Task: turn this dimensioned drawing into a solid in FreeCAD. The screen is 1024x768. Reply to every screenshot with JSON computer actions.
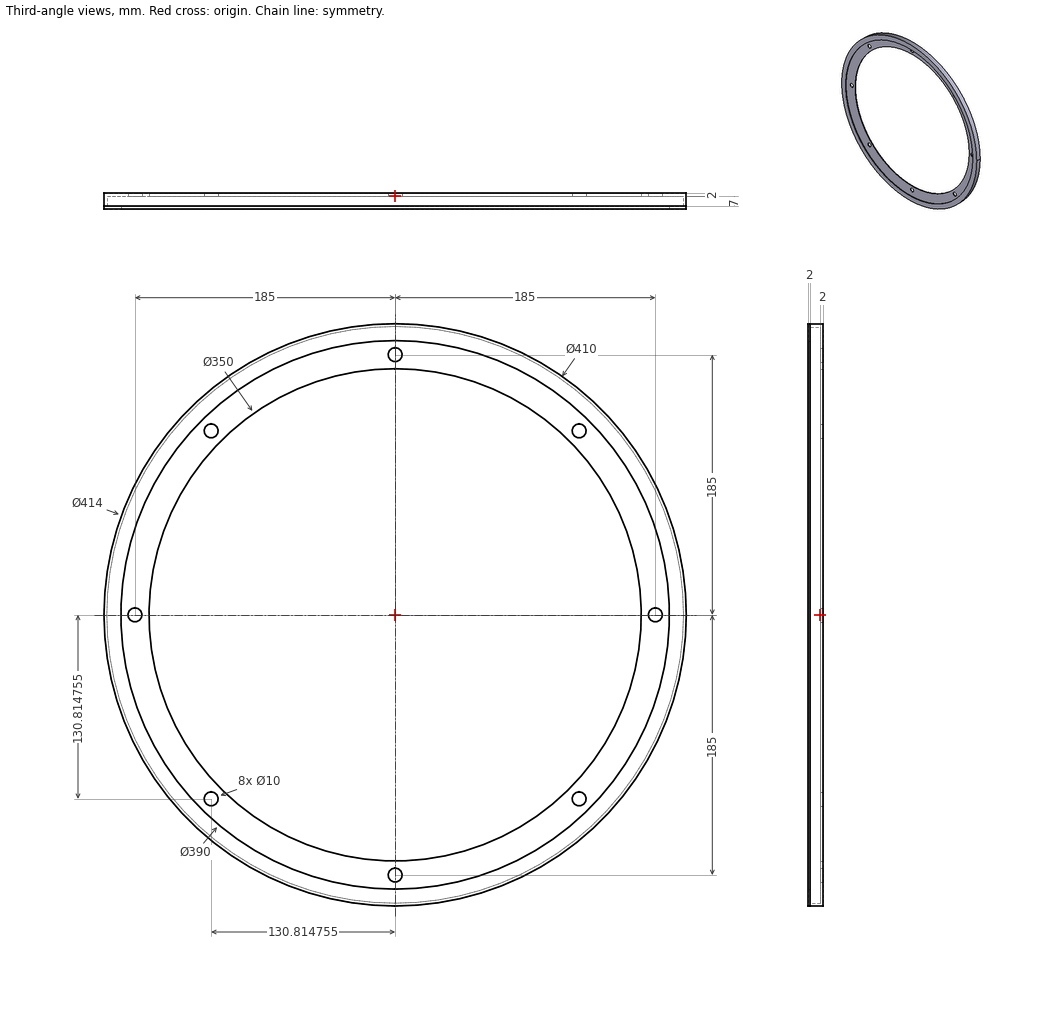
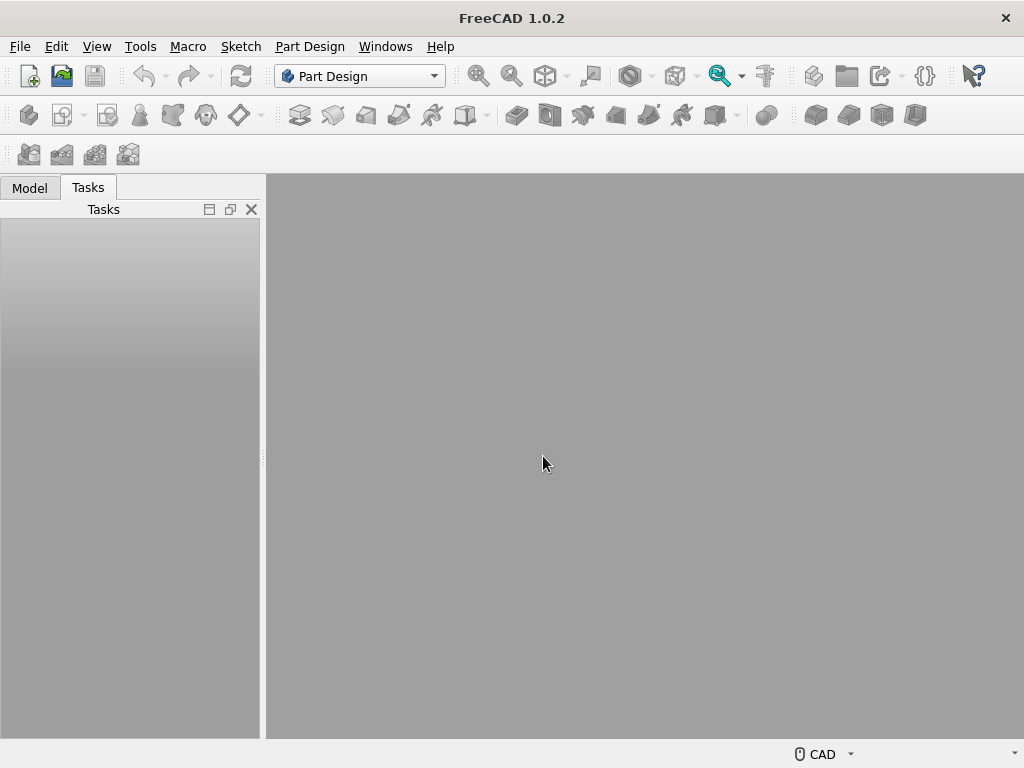
{"action": "left_click", "coordinate": [29, 76]}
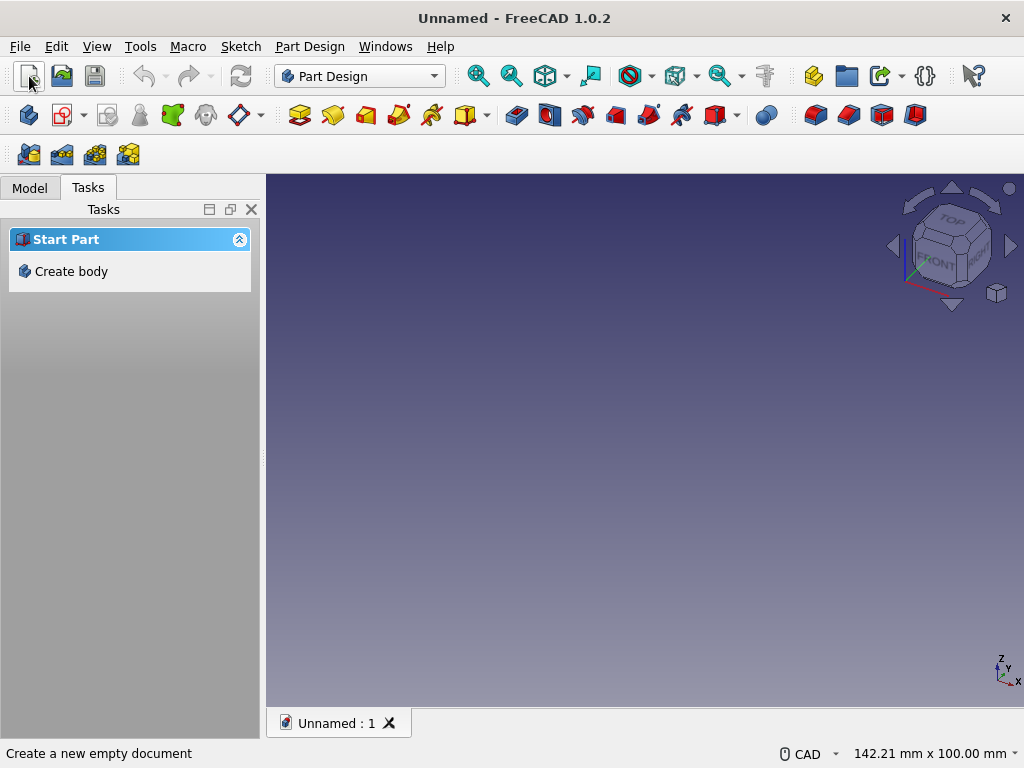
{"action": "left_click", "coordinate": [62, 116]}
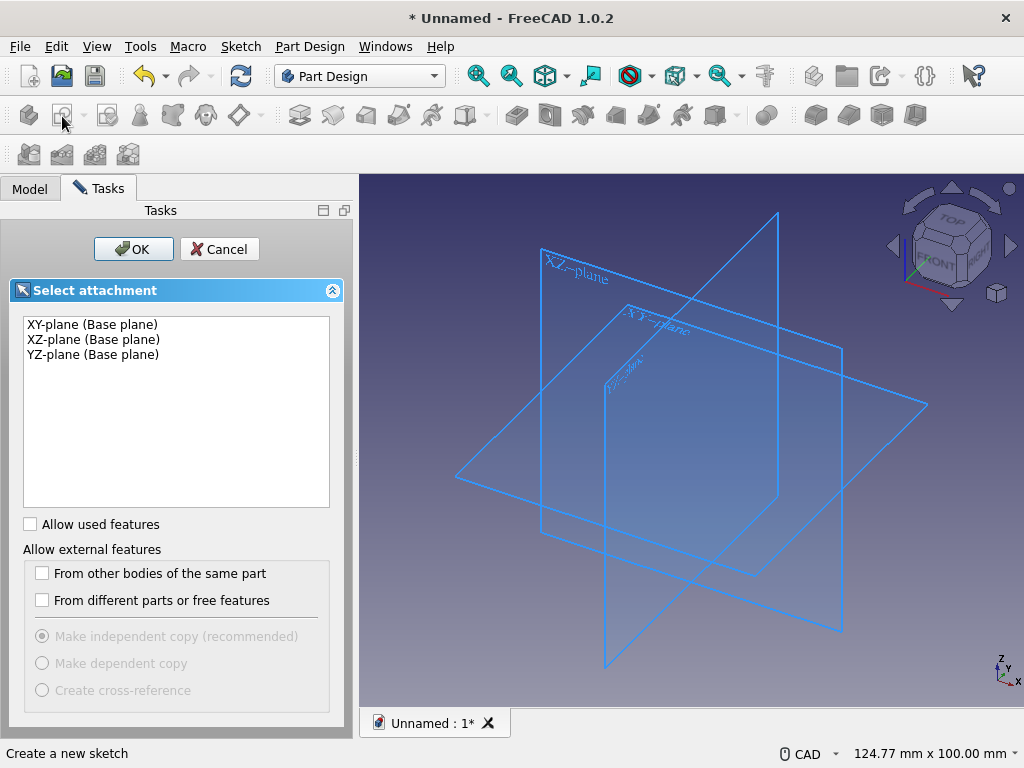
{"action": "left_click", "coordinate": [84, 340]}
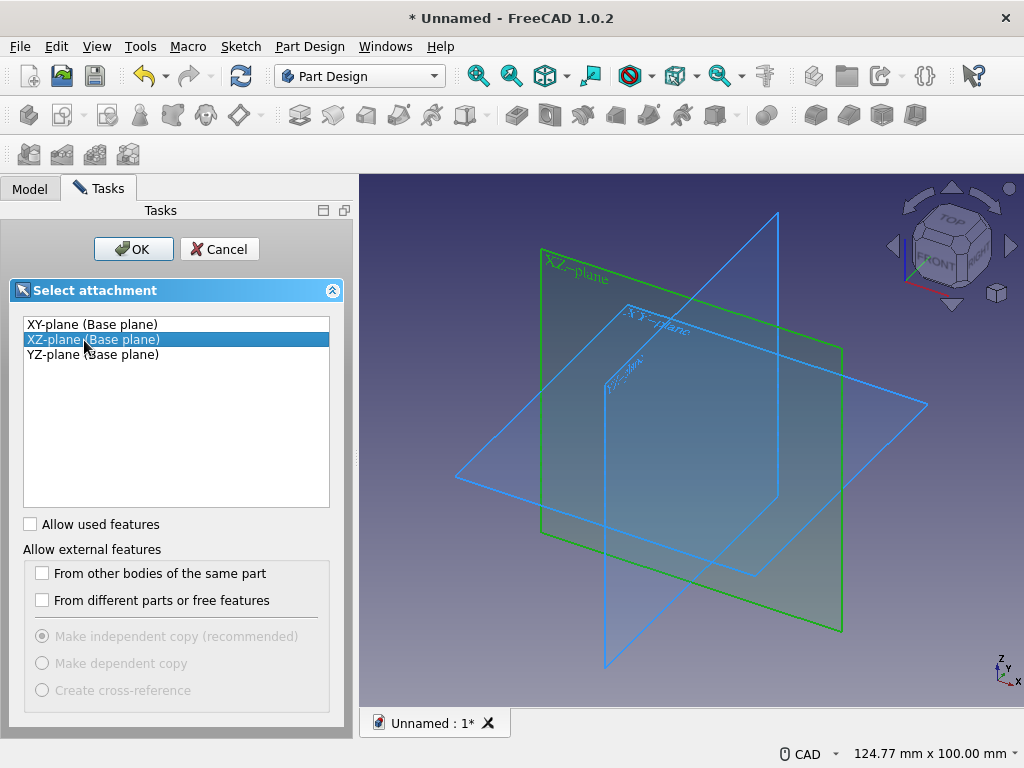
{"action": "left_click", "coordinate": [134, 249]}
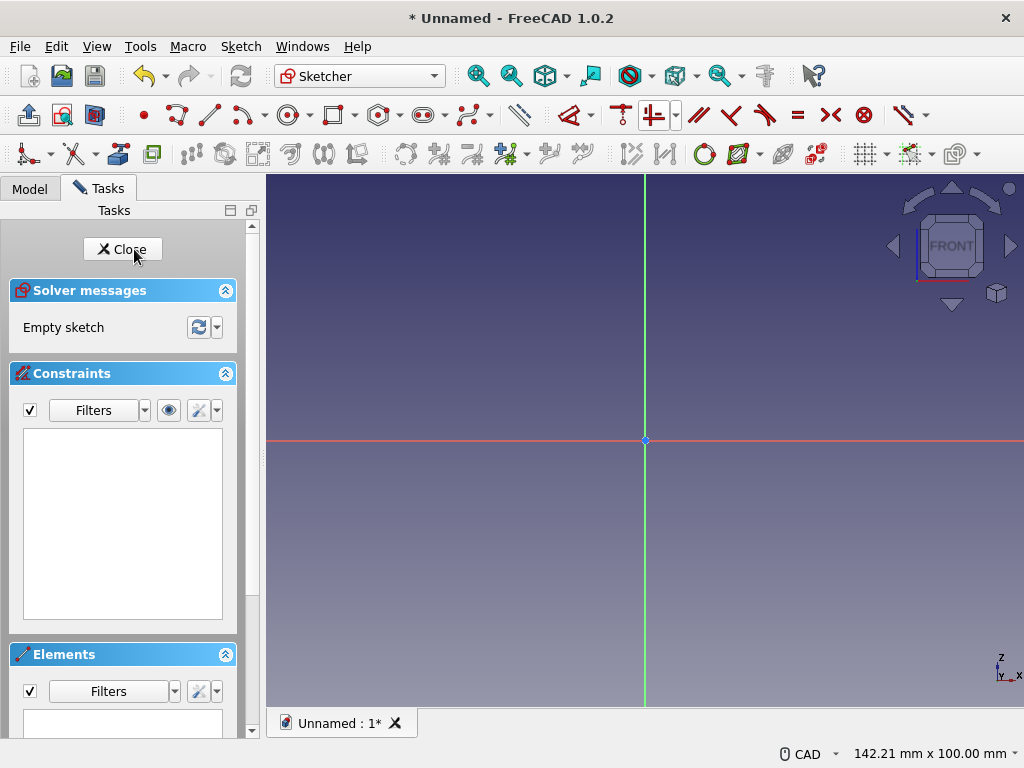
{"action": "scroll", "coordinate": [563, 440], "scroll_direction": "down", "scroll_amount": 9}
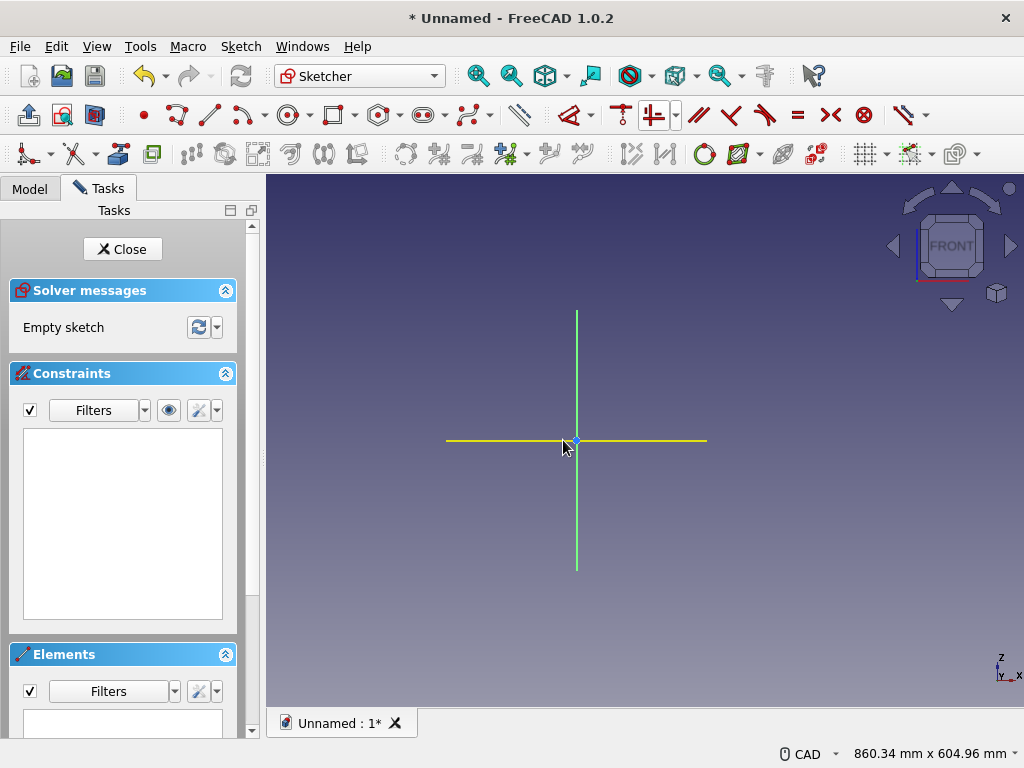
{"action": "left_click", "coordinate": [288, 116]}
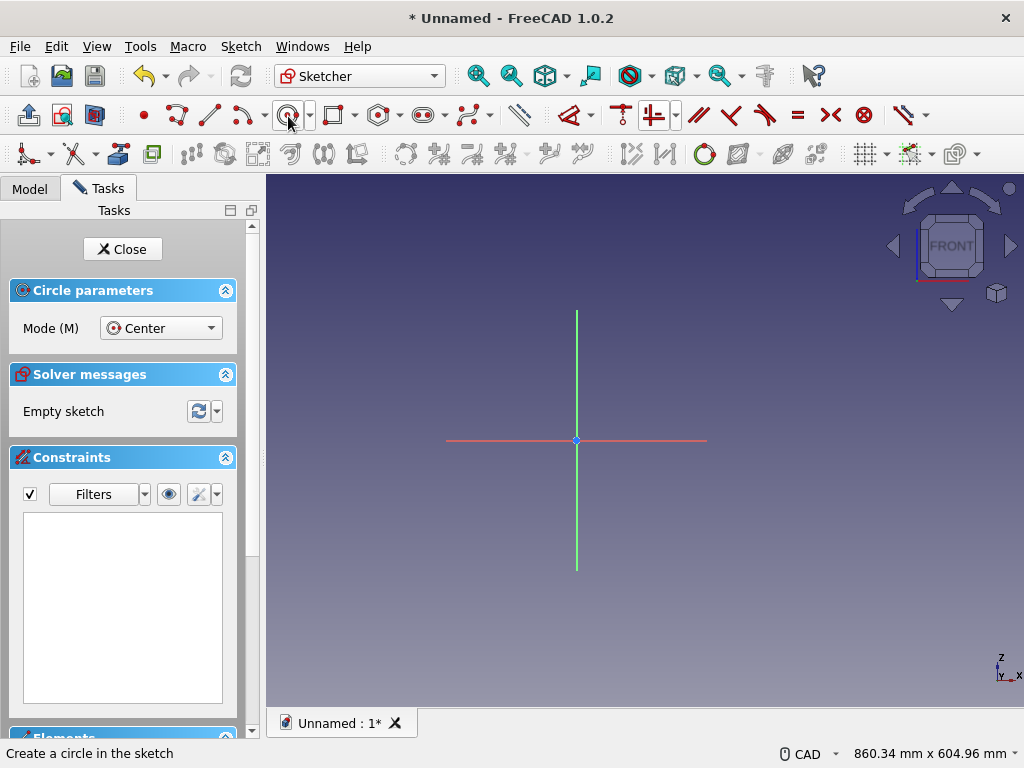
{"action": "left_click", "coordinate": [577, 440]}
{"action": "mouse_move", "coordinate": [705, 313]}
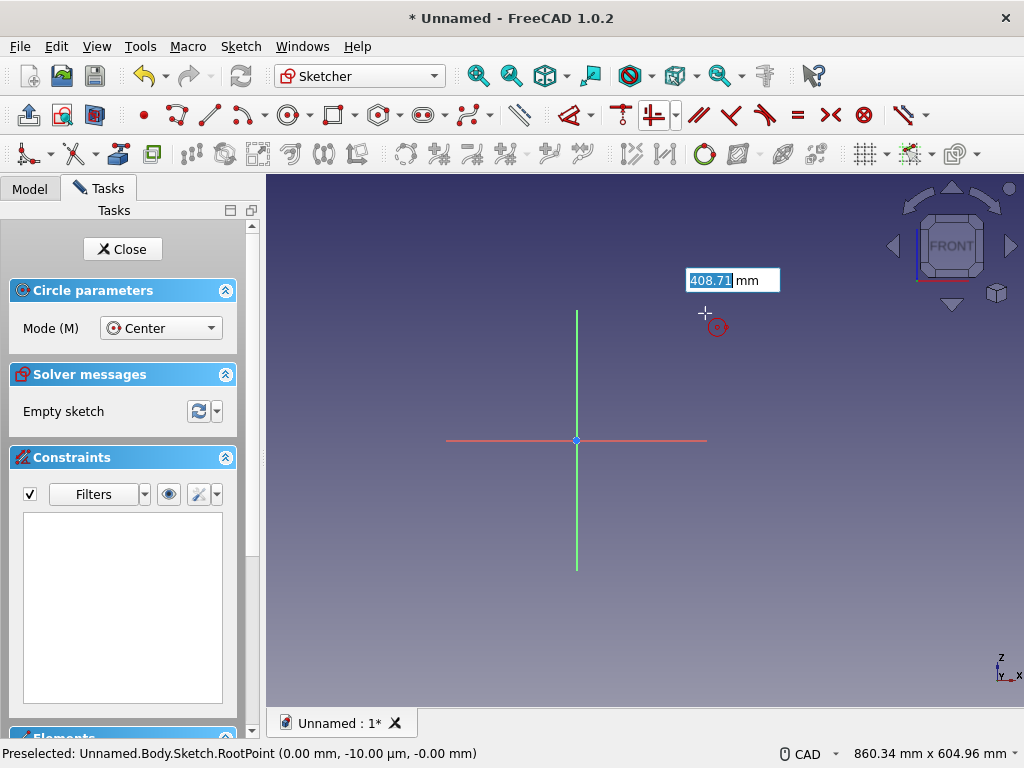
{"action": "type", "text": "410"}
{"action": "key", "text": "Return"}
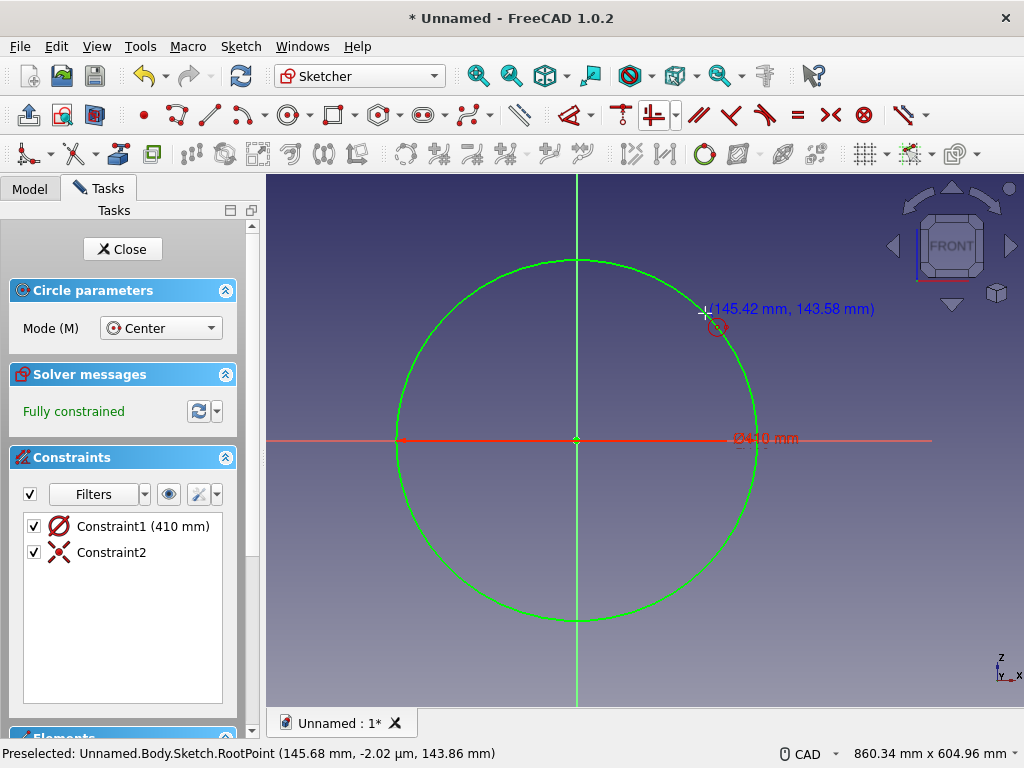
{"action": "scroll", "coordinate": [462, 556], "scroll_direction": "up", "scroll_amount": 9}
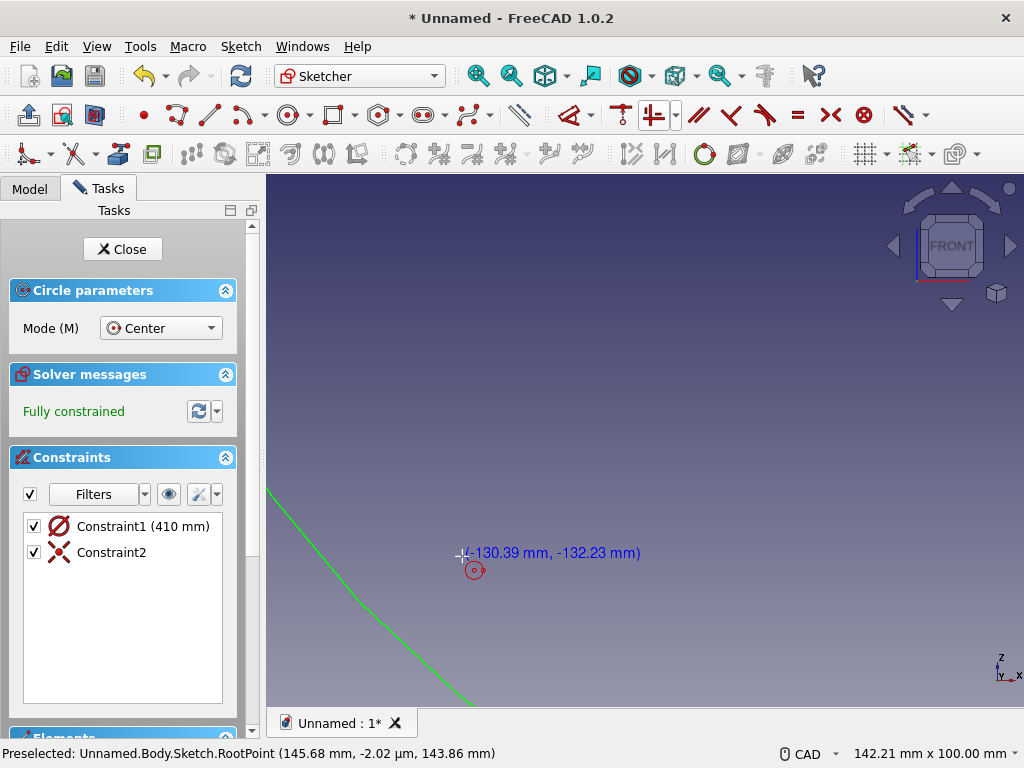
{"action": "scroll", "coordinate": [462, 557], "scroll_direction": "down", "scroll_amount": 9}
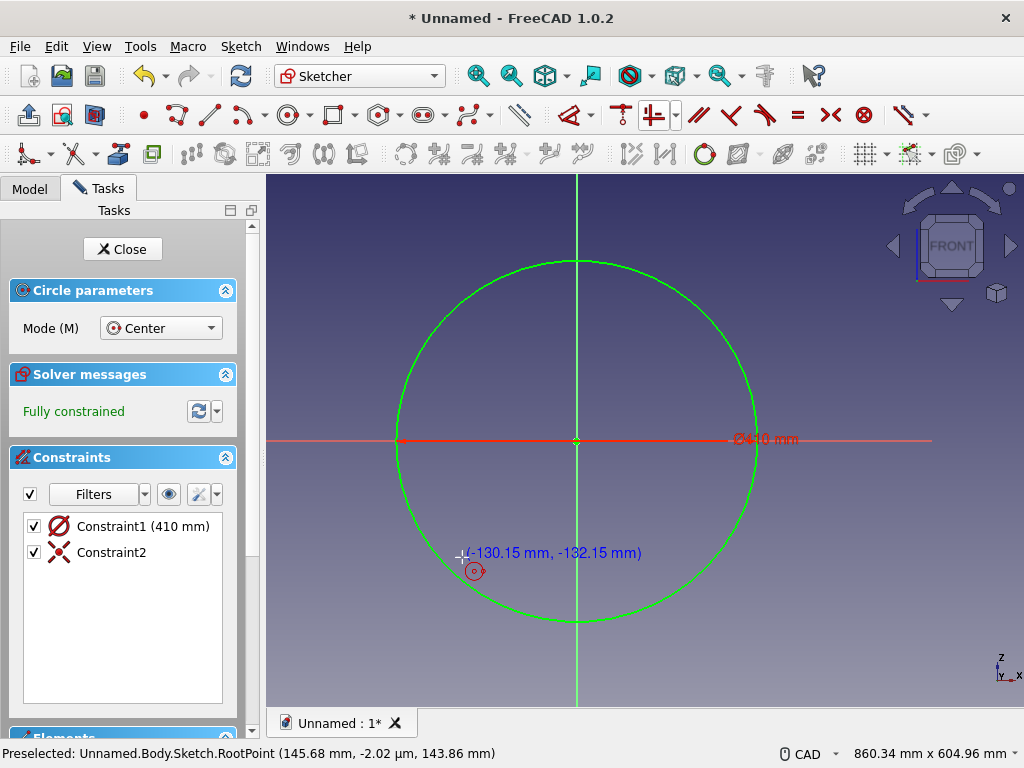
{"action": "left_click", "coordinate": [462, 557]}
{"action": "mouse_move", "coordinate": [465, 553]}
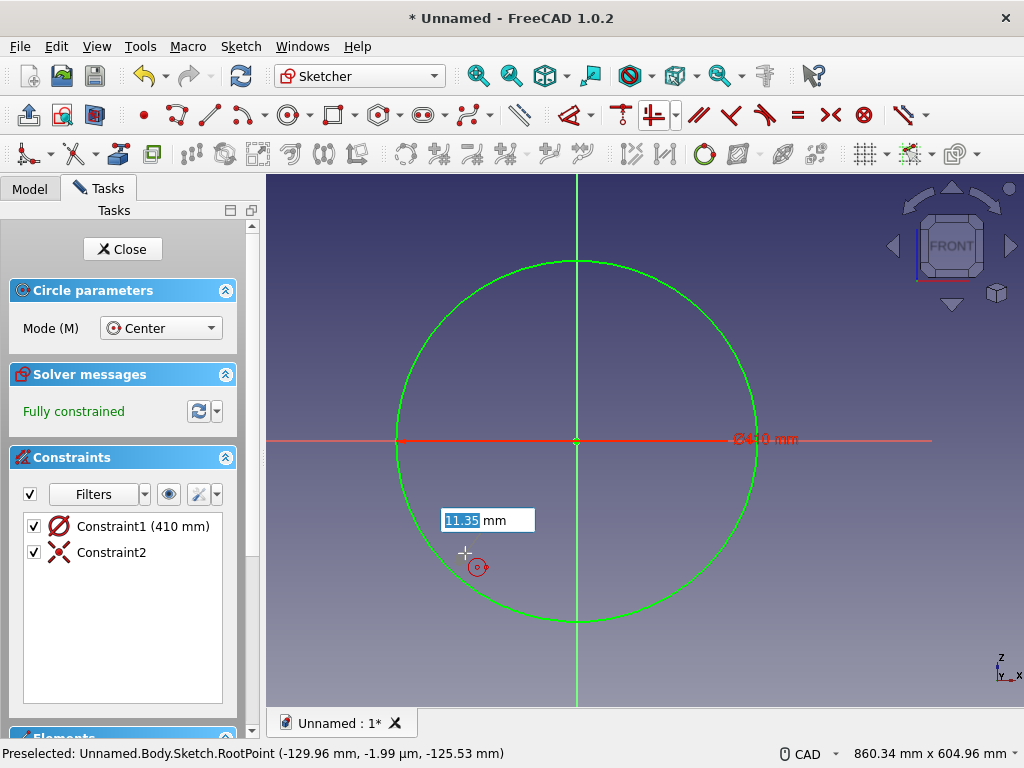
{"action": "type", "text": "10"}
{"action": "key", "text": "Return"}